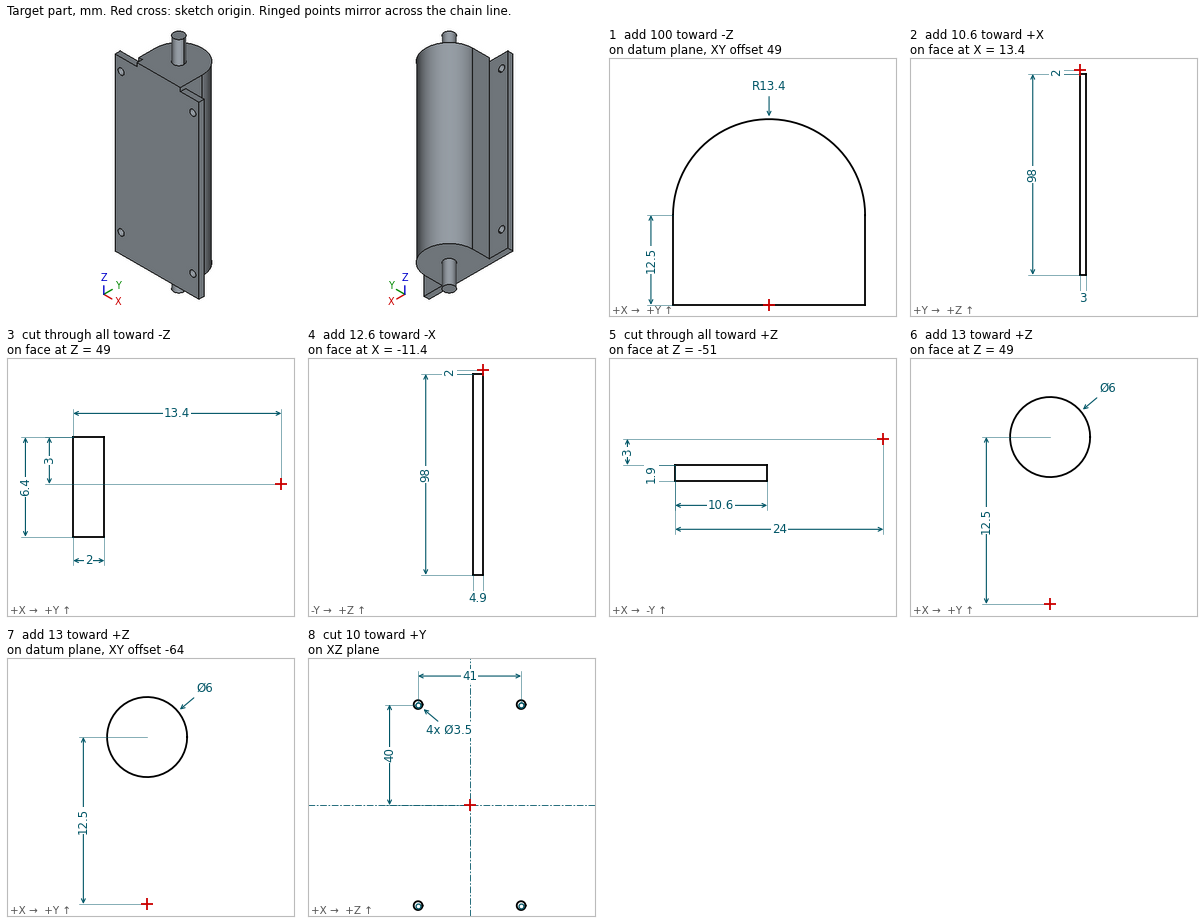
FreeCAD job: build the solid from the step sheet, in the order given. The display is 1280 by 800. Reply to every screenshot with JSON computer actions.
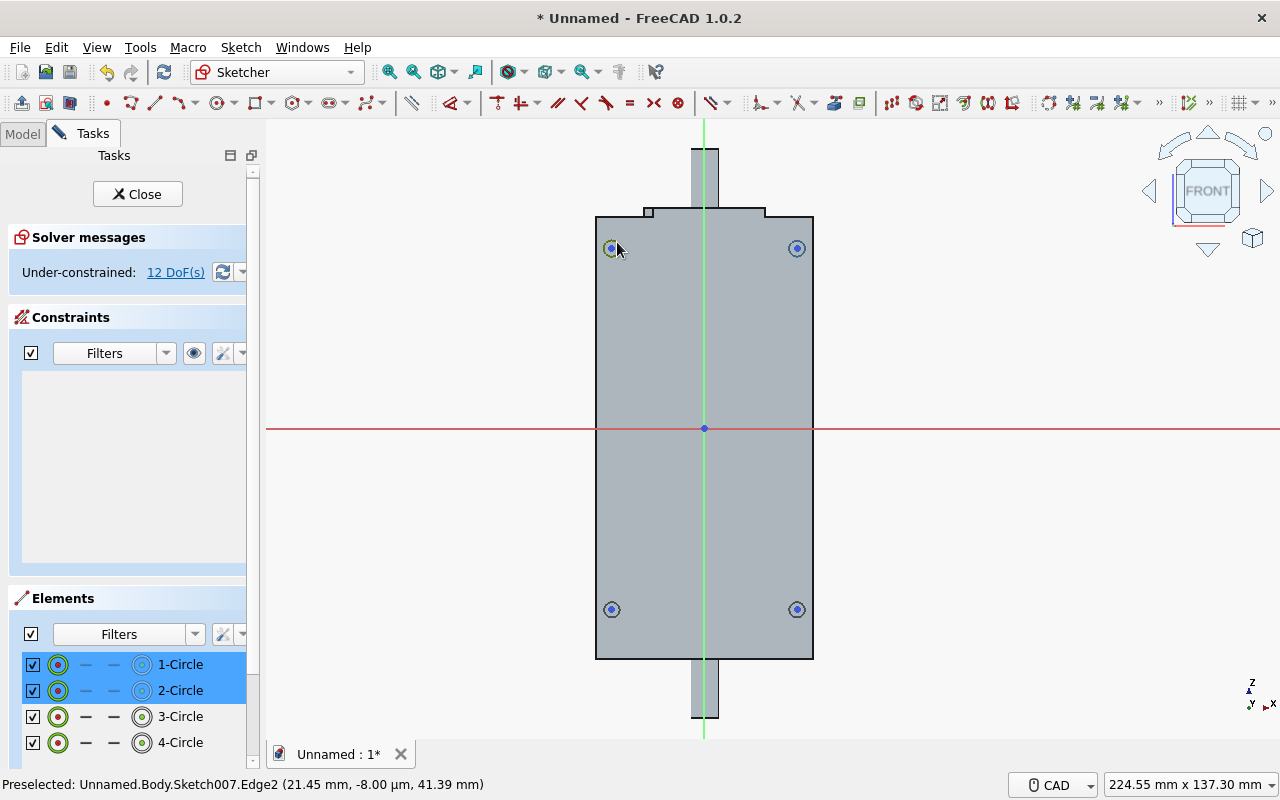
{"action": "scroll", "coordinate": [802, 604], "scroll_direction": "up", "scroll_amount": 3}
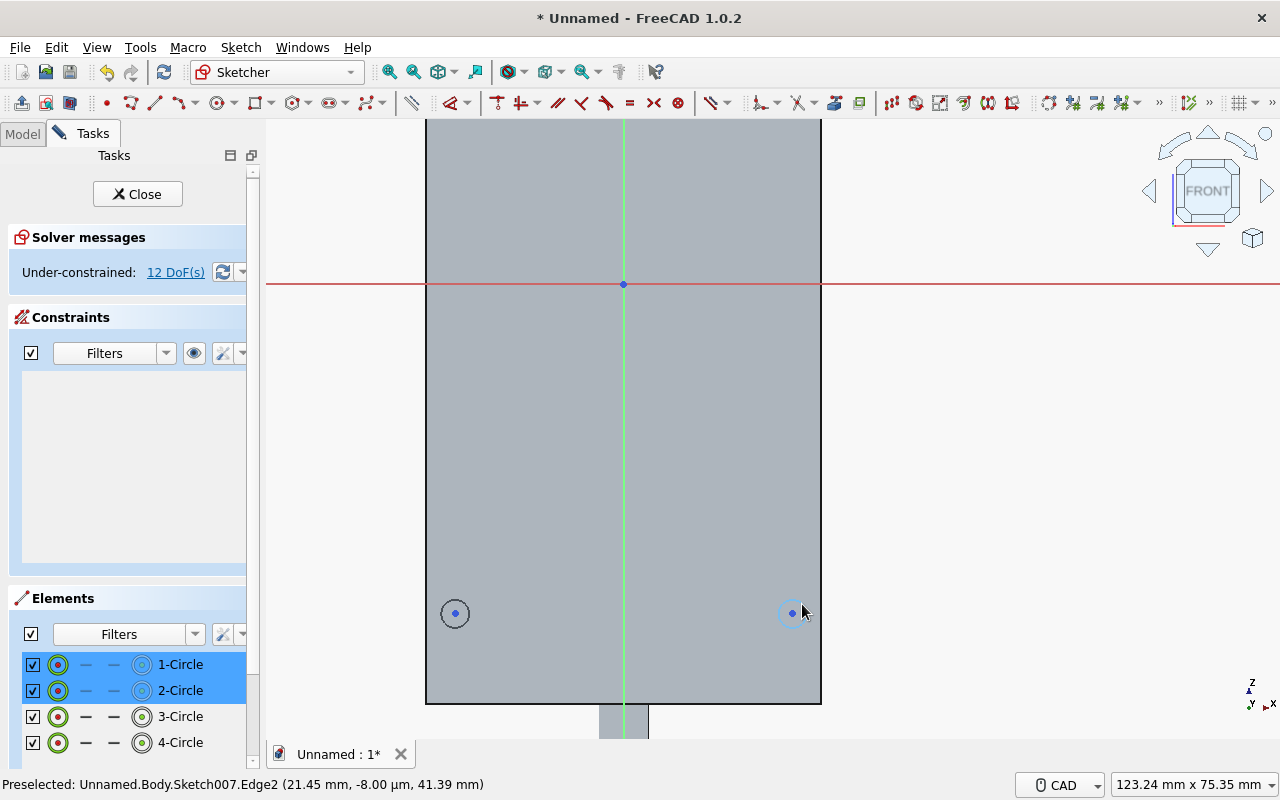
{"action": "left_click", "coordinate": [802, 604]}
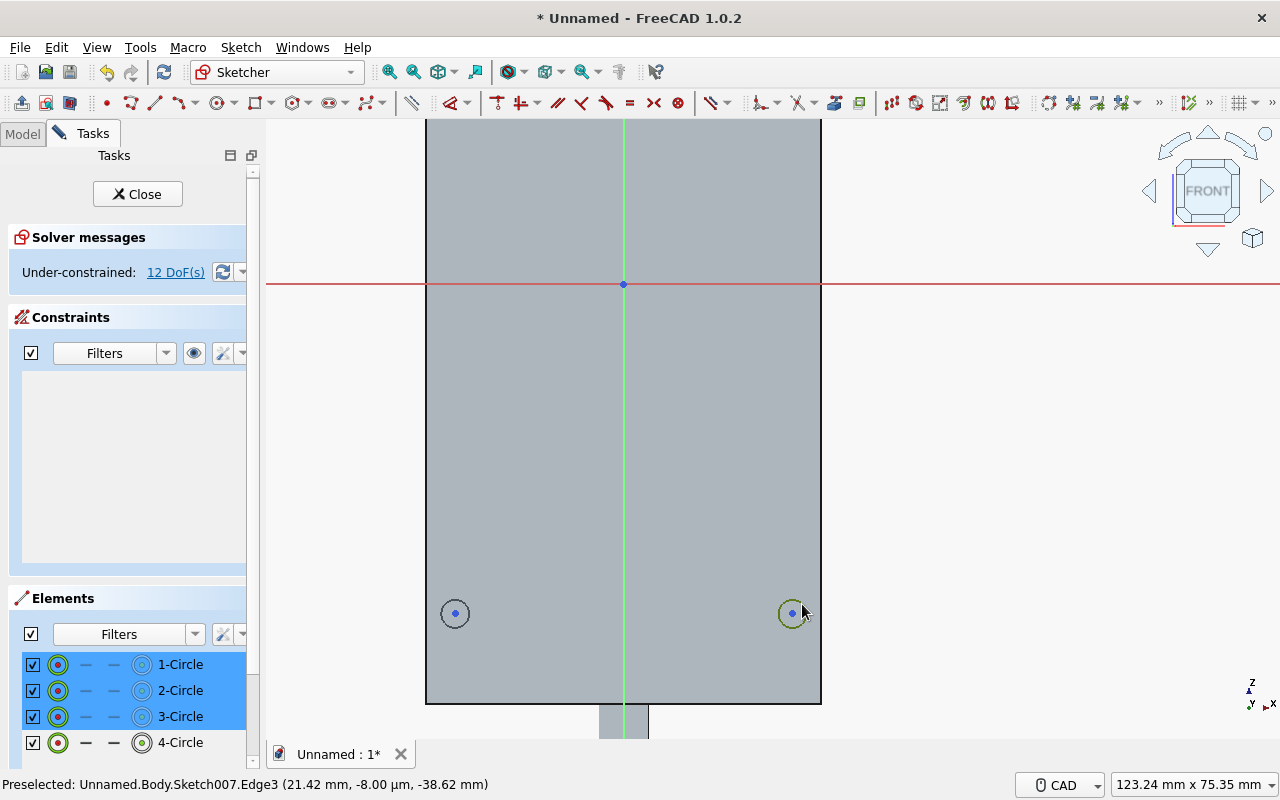
{"action": "left_click", "coordinate": [465, 604]}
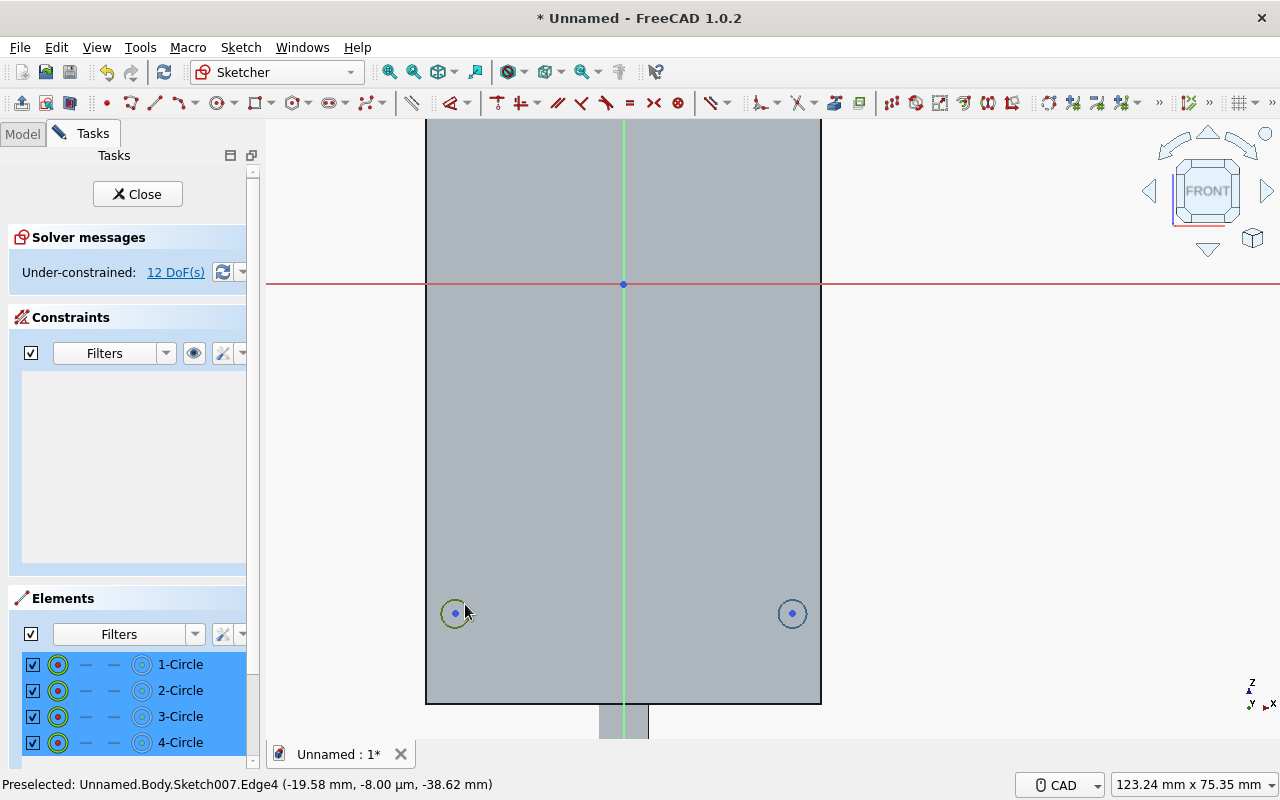
{"action": "left_click", "coordinate": [630, 104]}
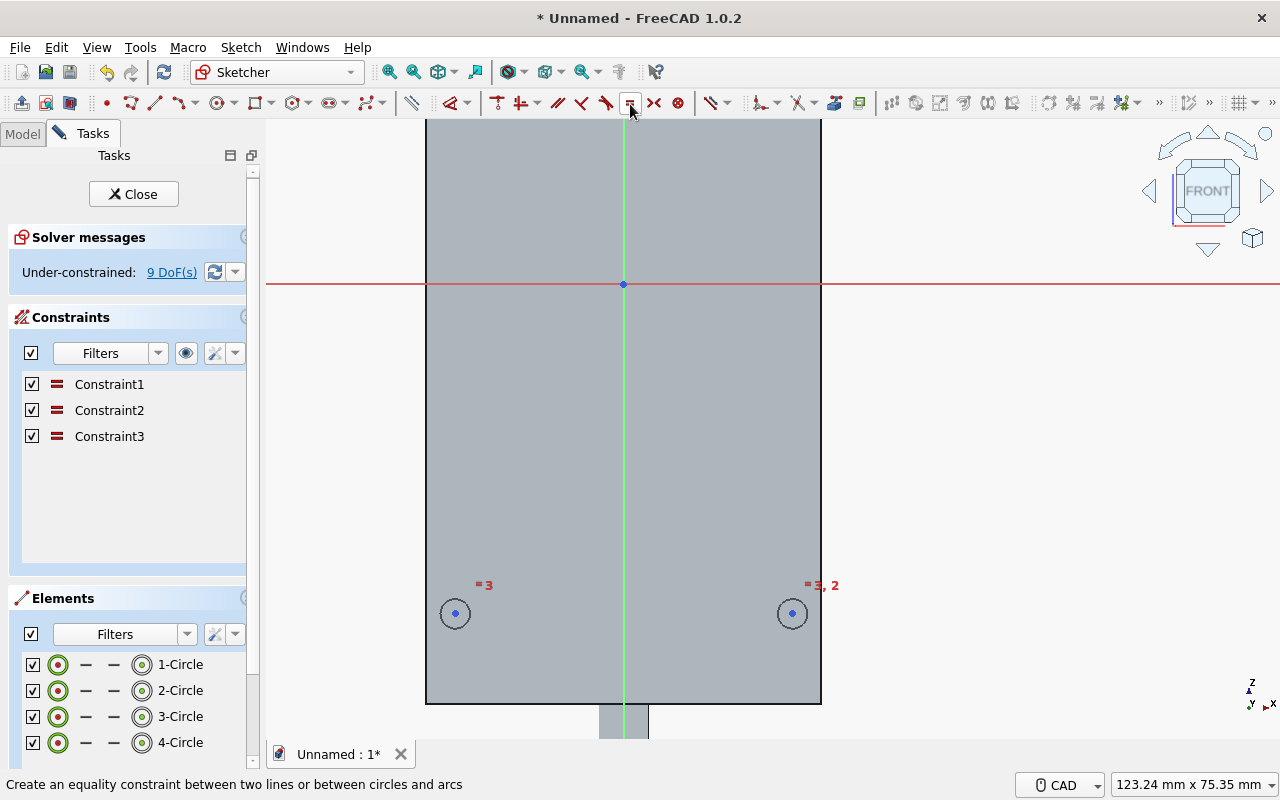
{"action": "scroll", "coordinate": [803, 605], "scroll_direction": "down", "scroll_amount": 3}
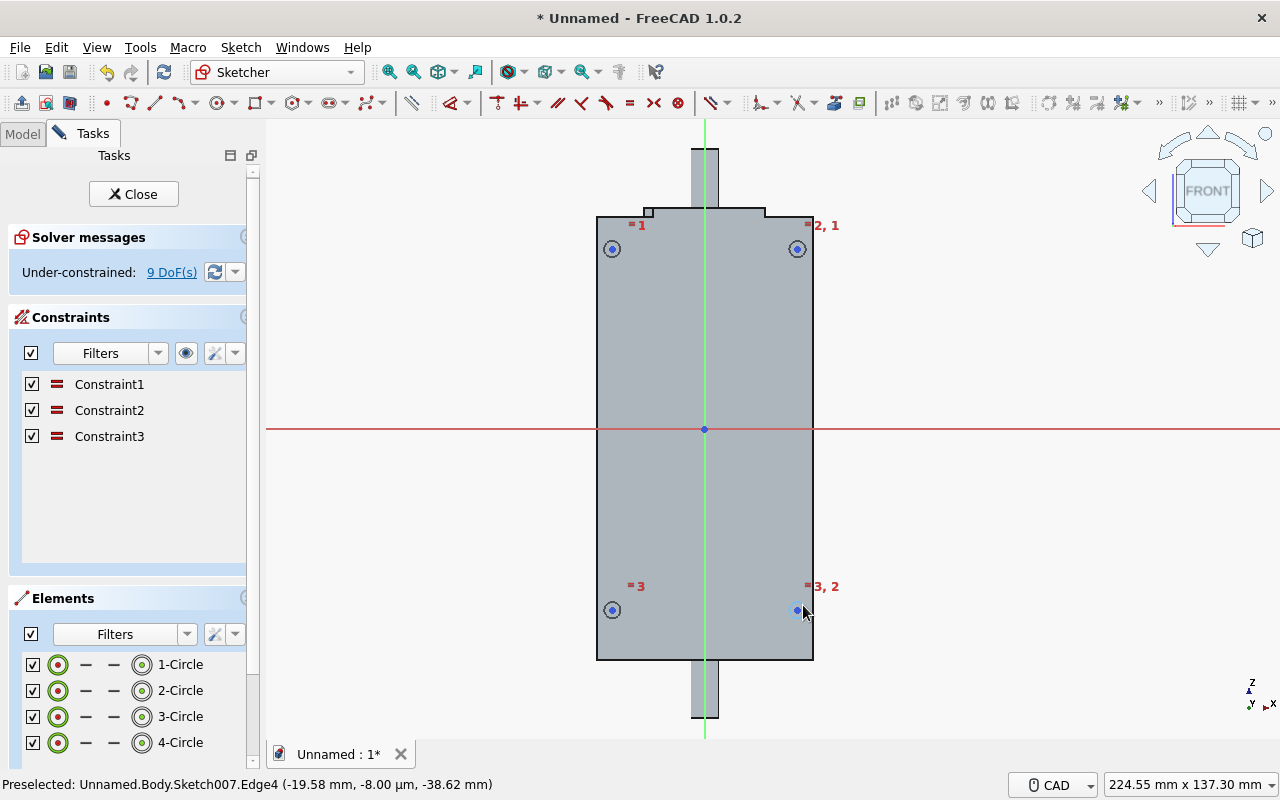
{"action": "left_click", "coordinate": [612, 249]}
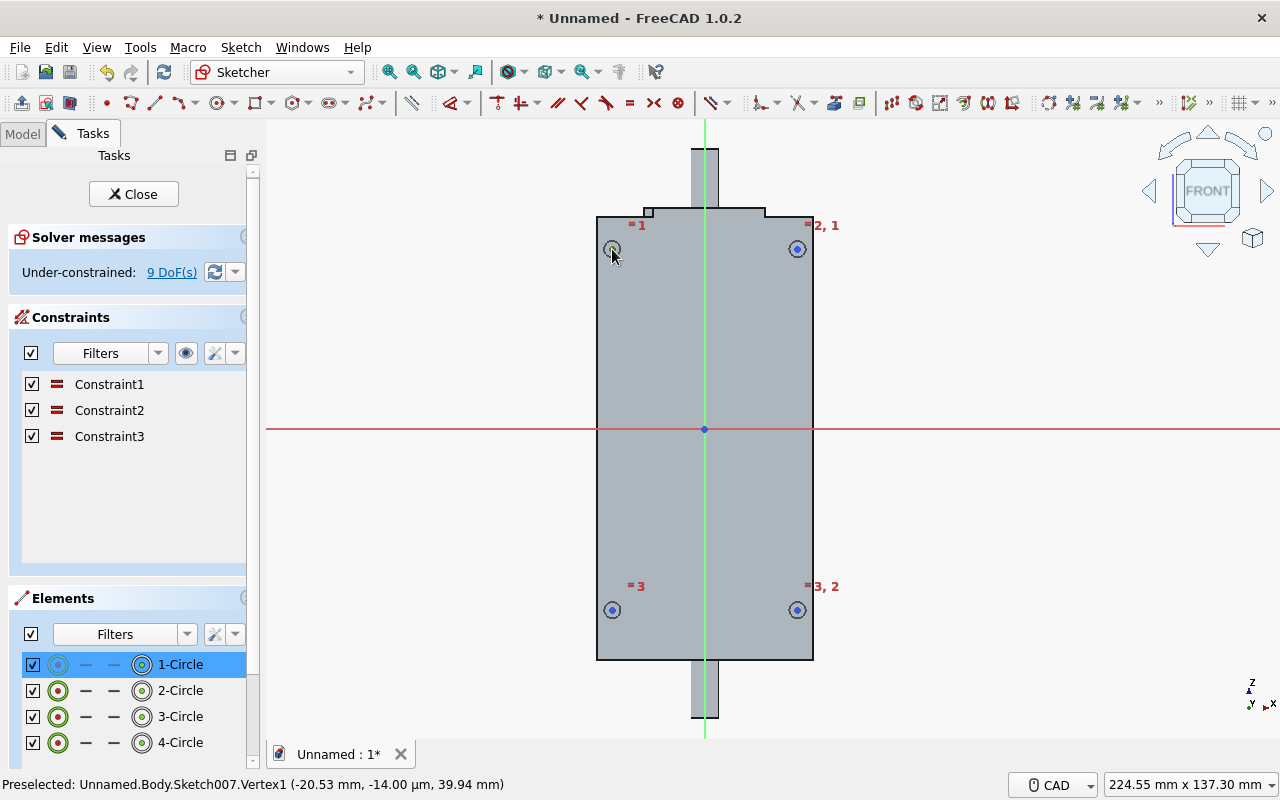
{"action": "left_click", "coordinate": [798, 249]}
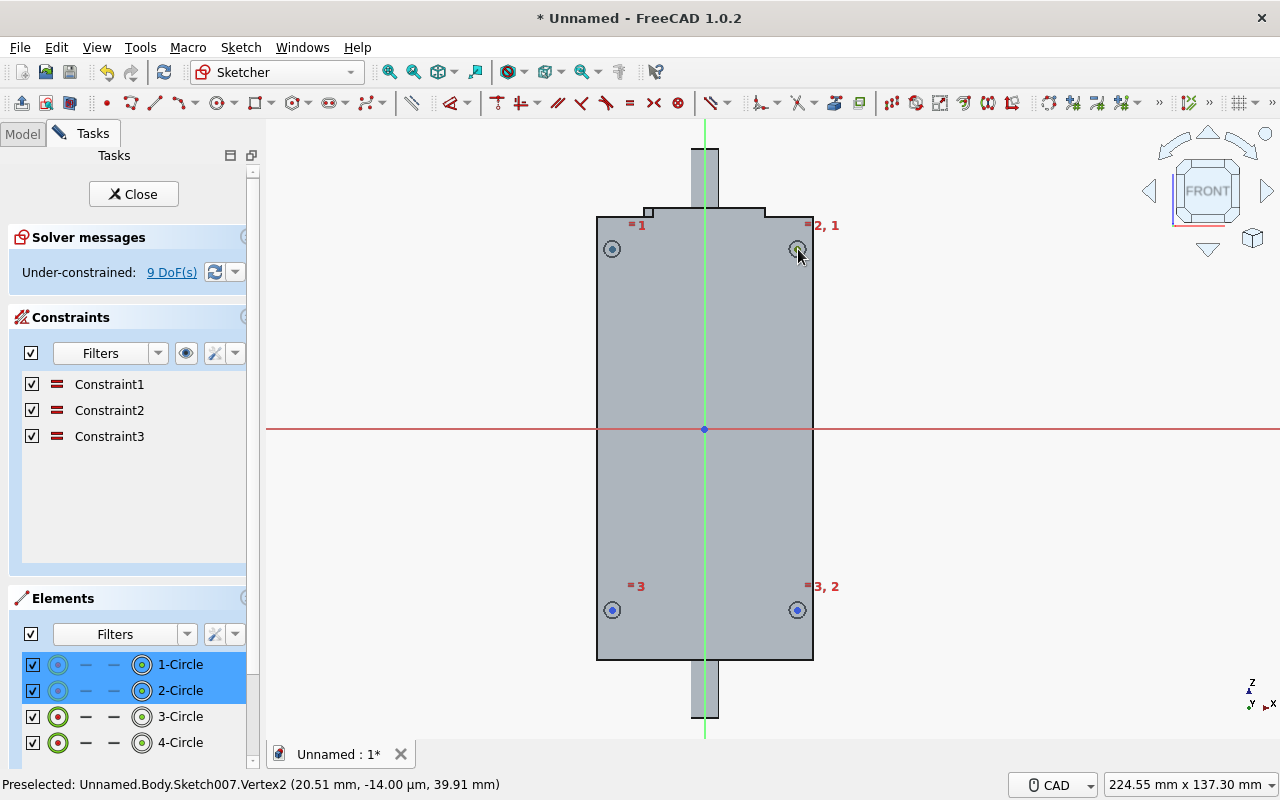
{"action": "left_click", "coordinate": [705, 671]}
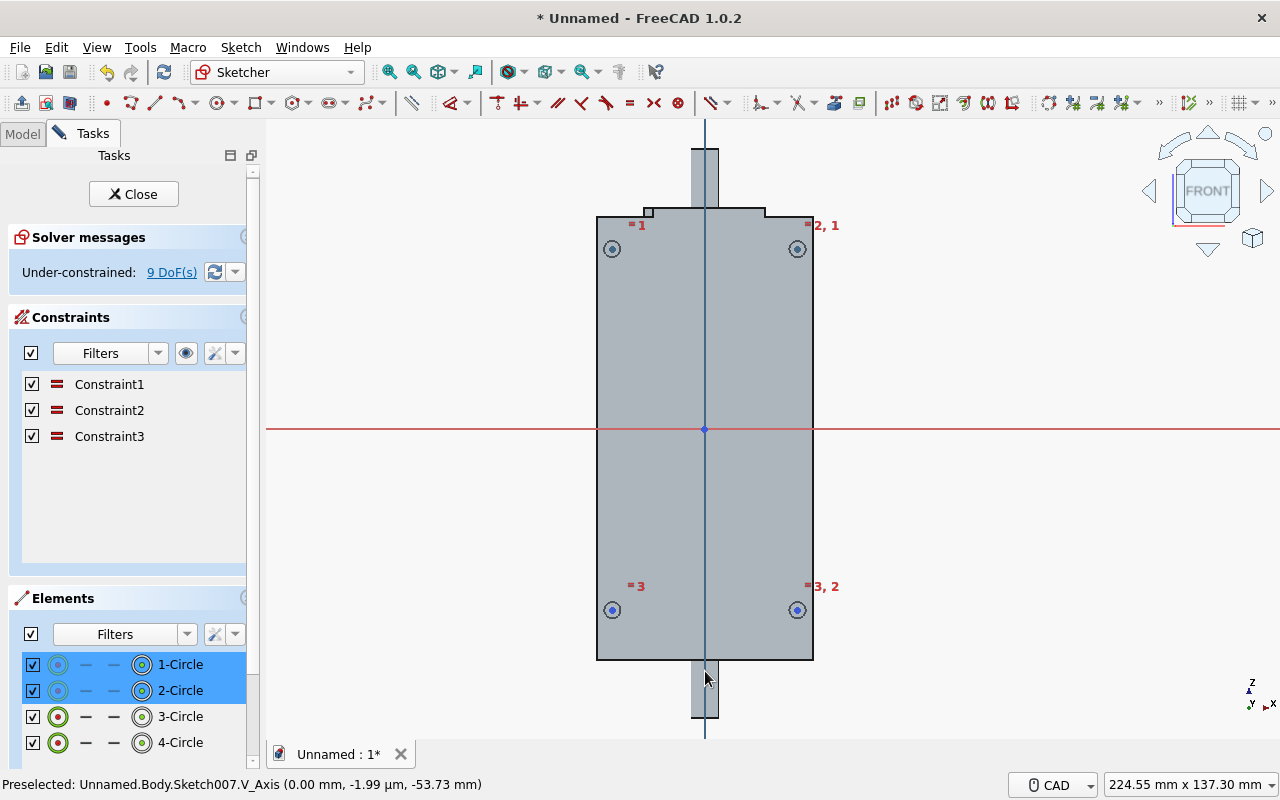
{"action": "left_click", "coordinate": [654, 104]}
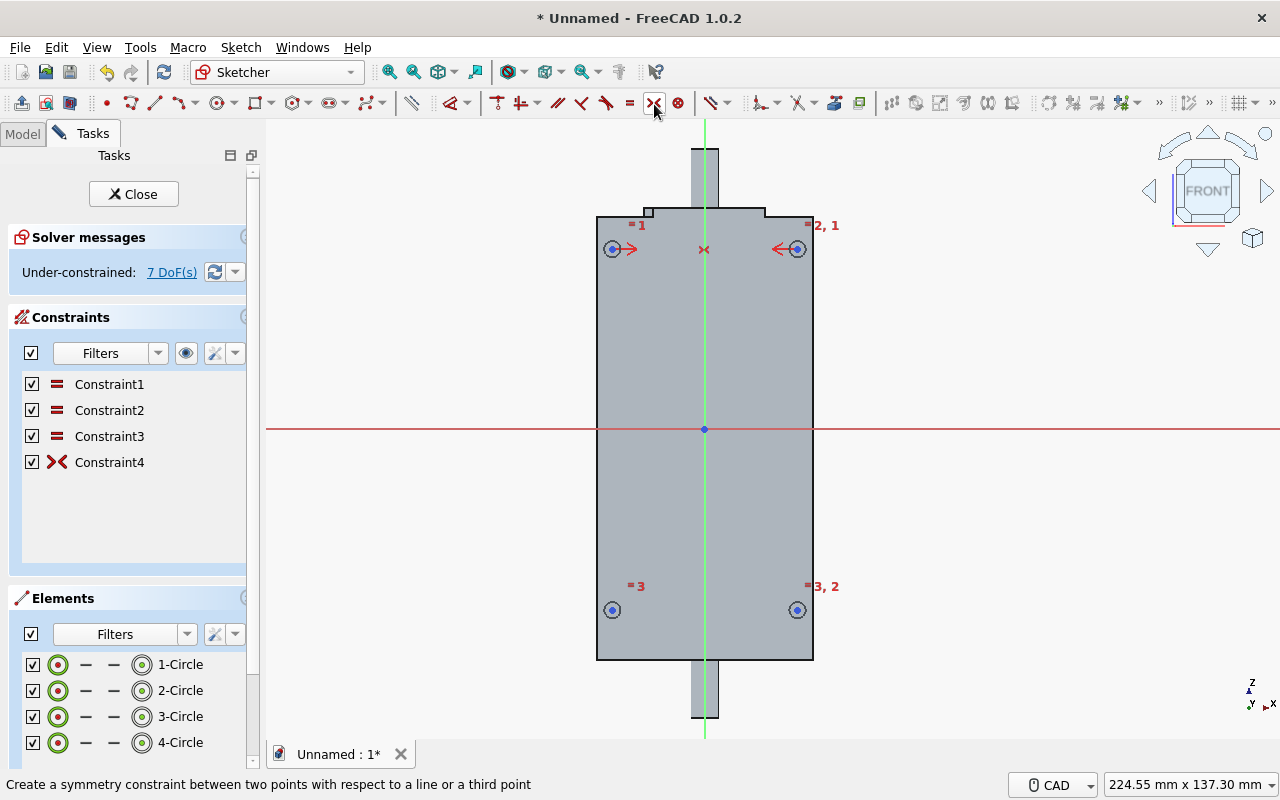
{"action": "left_click", "coordinate": [798, 249]}